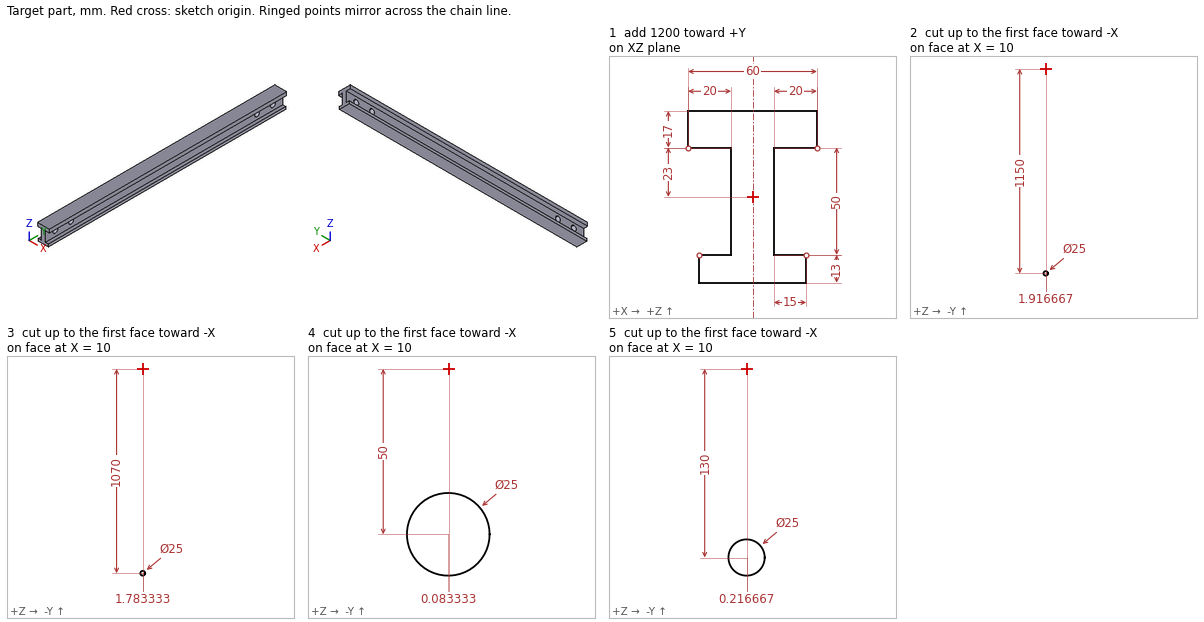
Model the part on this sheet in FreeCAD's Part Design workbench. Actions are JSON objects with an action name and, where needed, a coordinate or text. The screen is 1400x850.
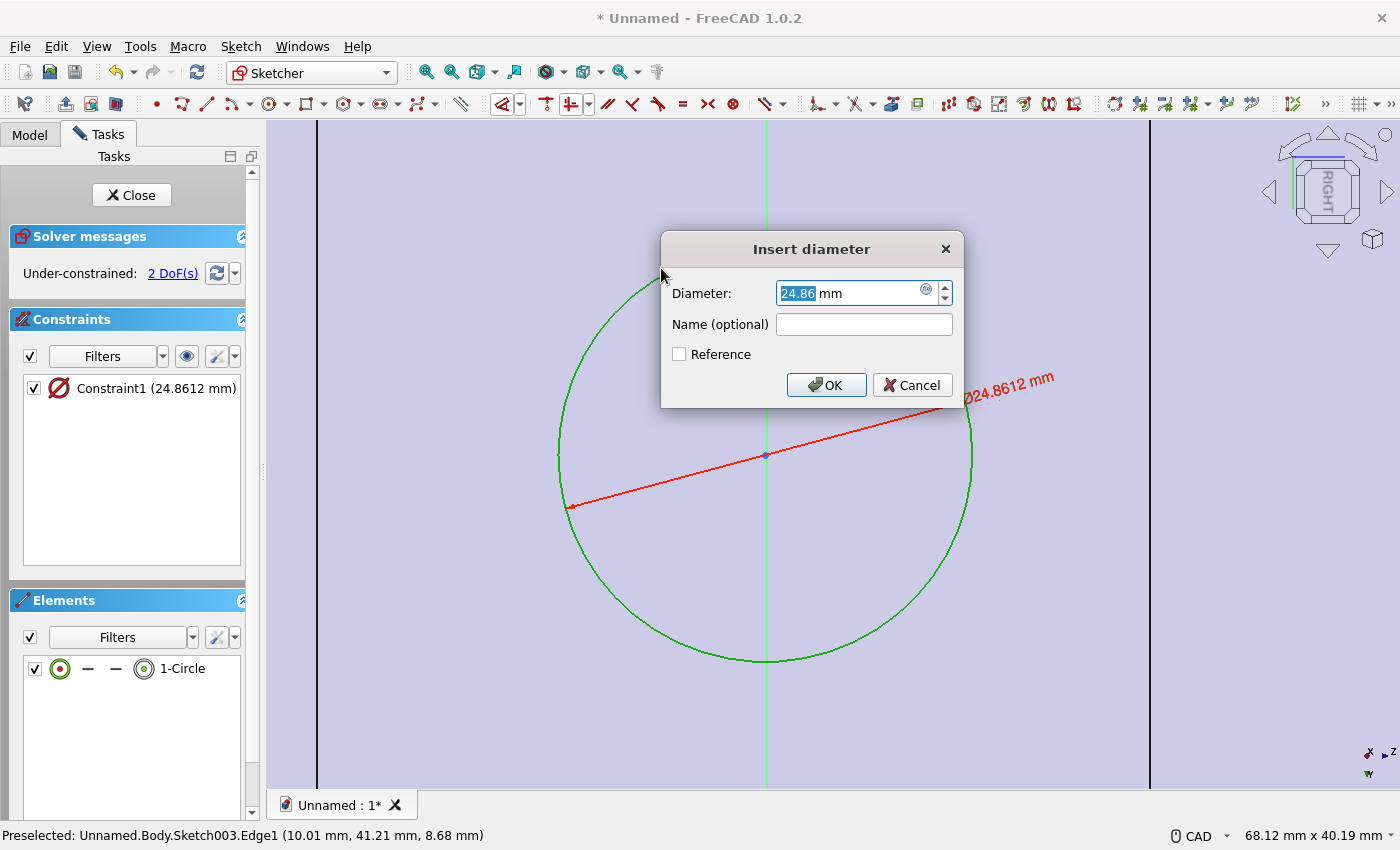
{"action": "type", "text": "25"}
{"action": "key", "text": "Return"}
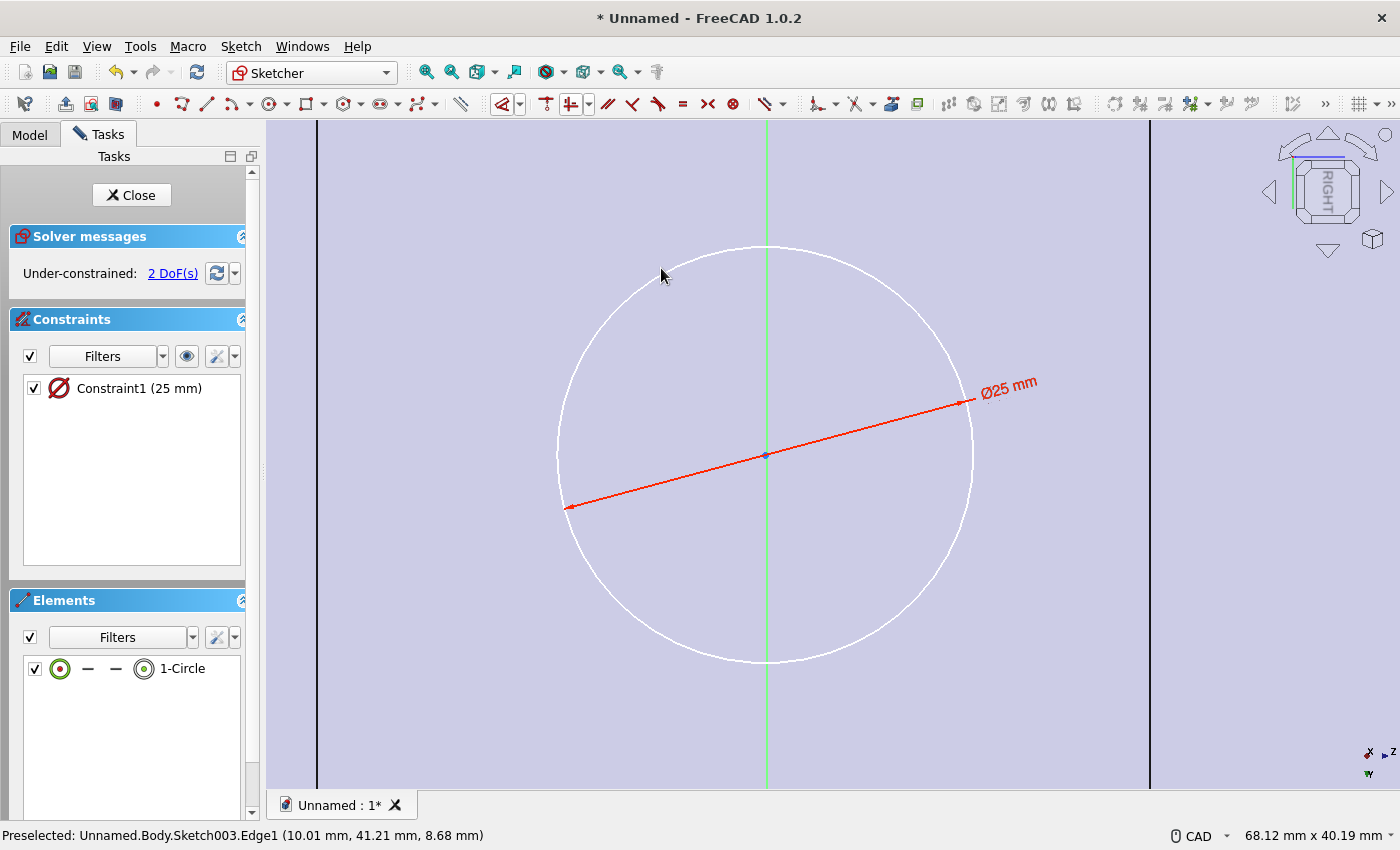
{"action": "left_click", "coordinate": [765, 455]}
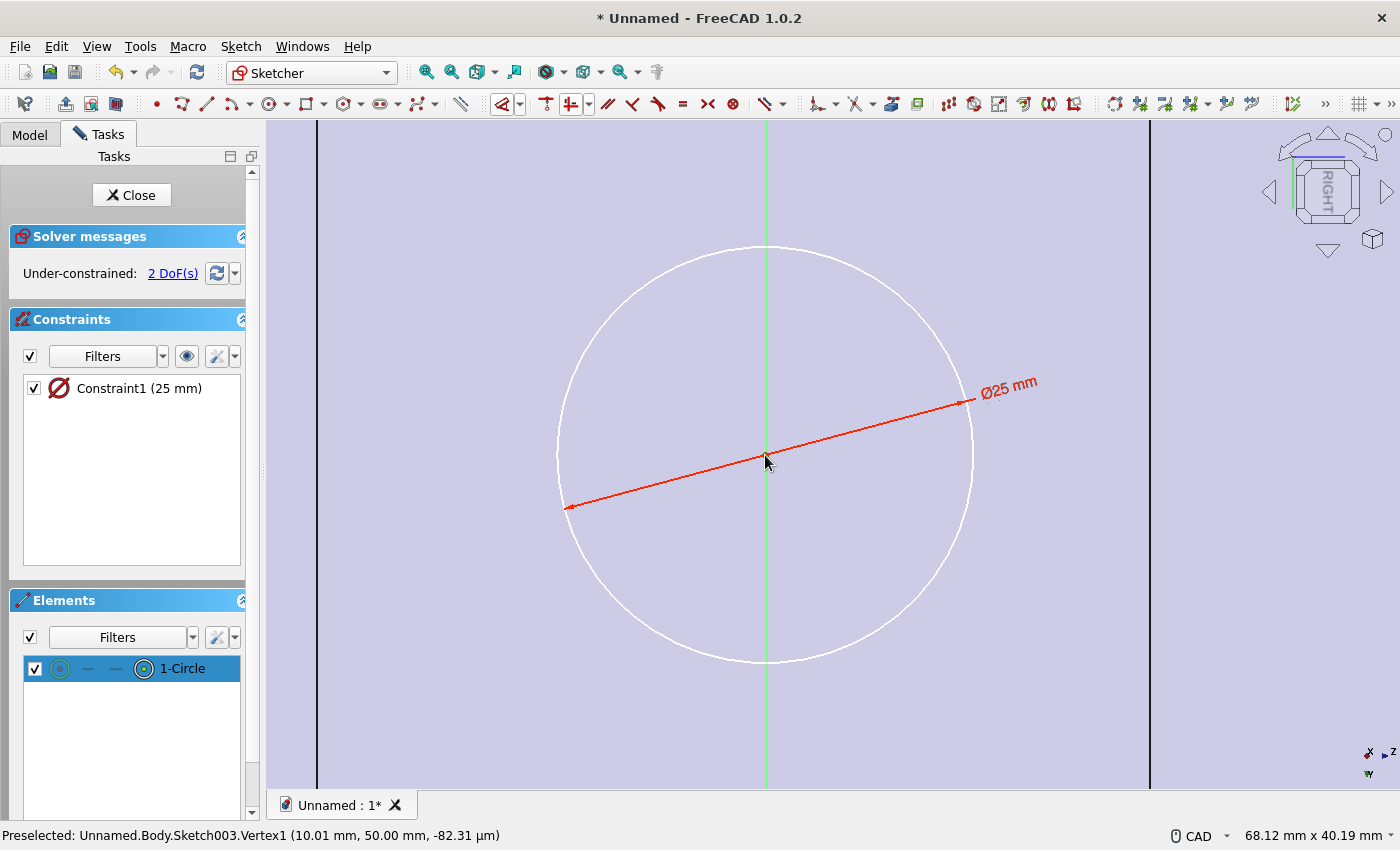
{"action": "left_click", "coordinate": [520, 104]}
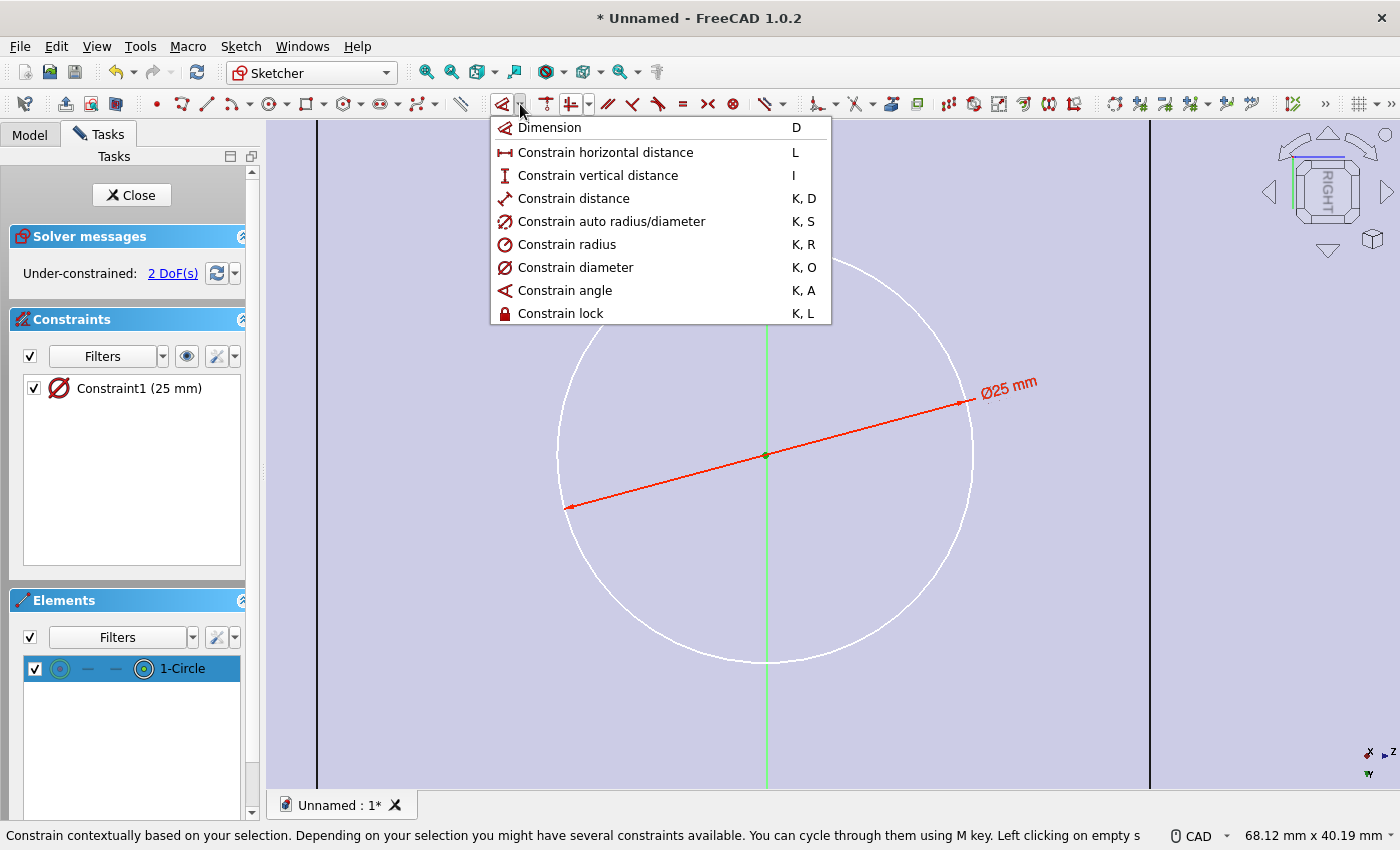
{"action": "left_click", "coordinate": [661, 176]}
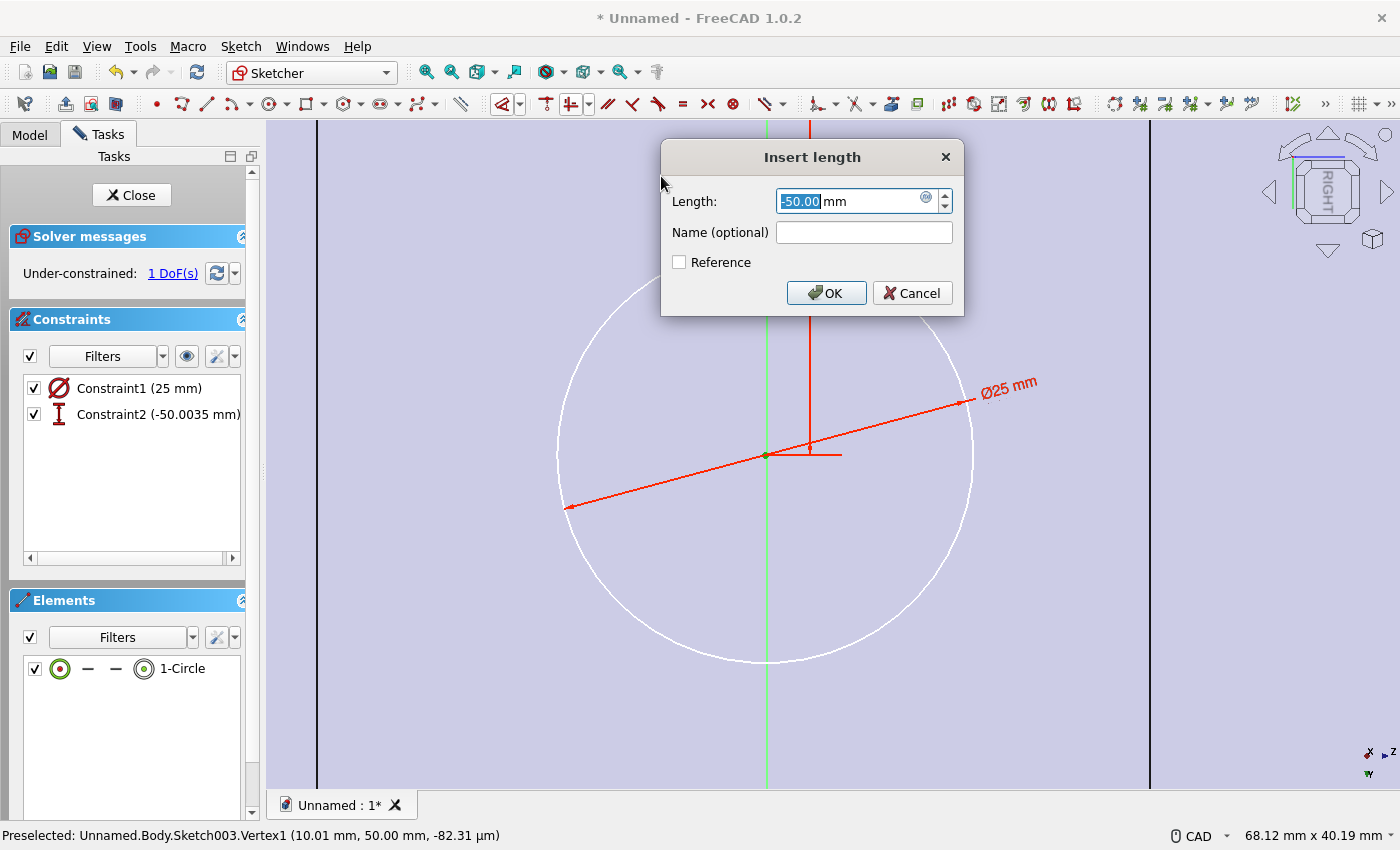
{"action": "type", "text": "-50"}
{"action": "key", "text": "Return"}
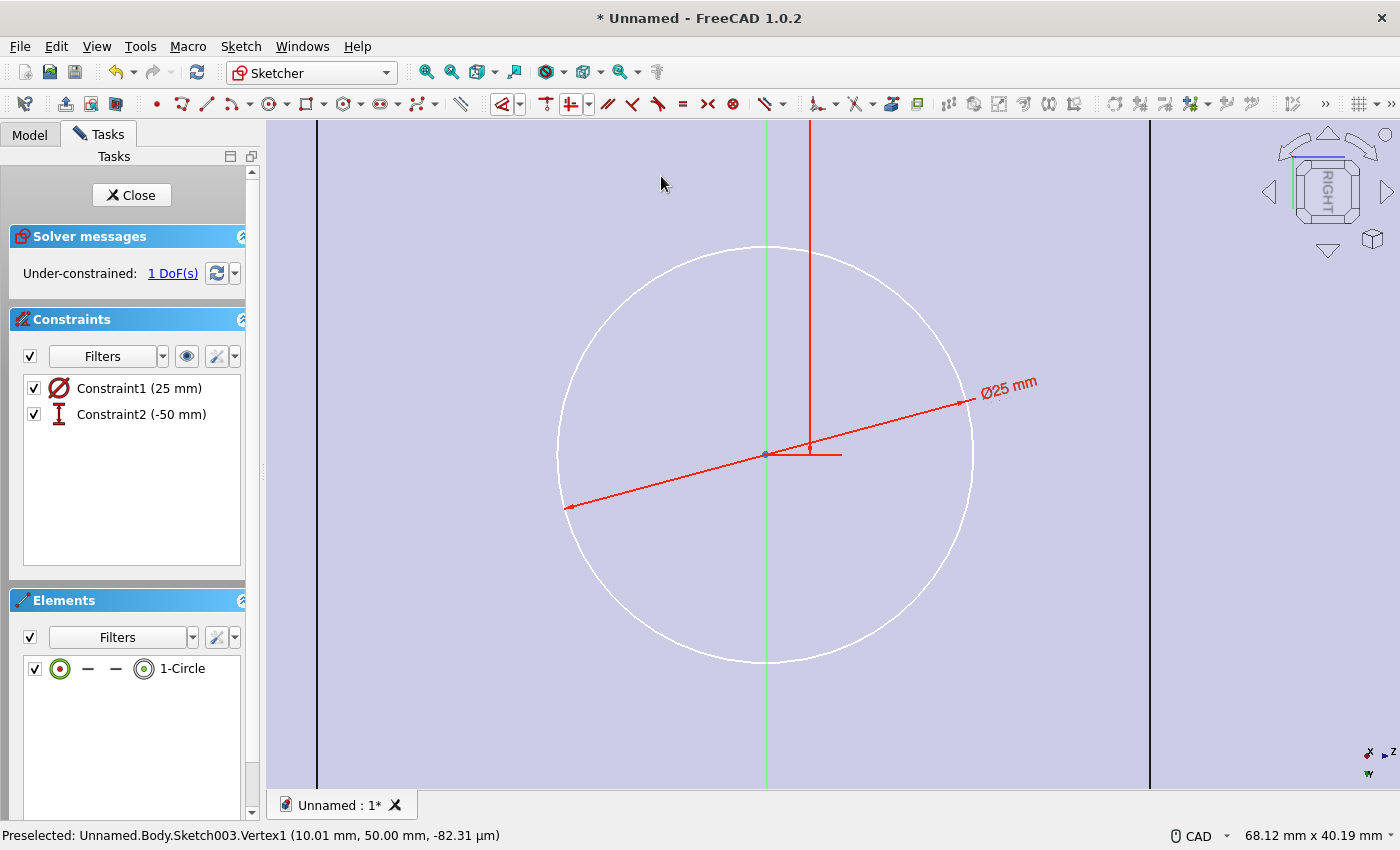
{"action": "scroll", "coordinate": [765, 455], "scroll_direction": "up", "scroll_amount": 17}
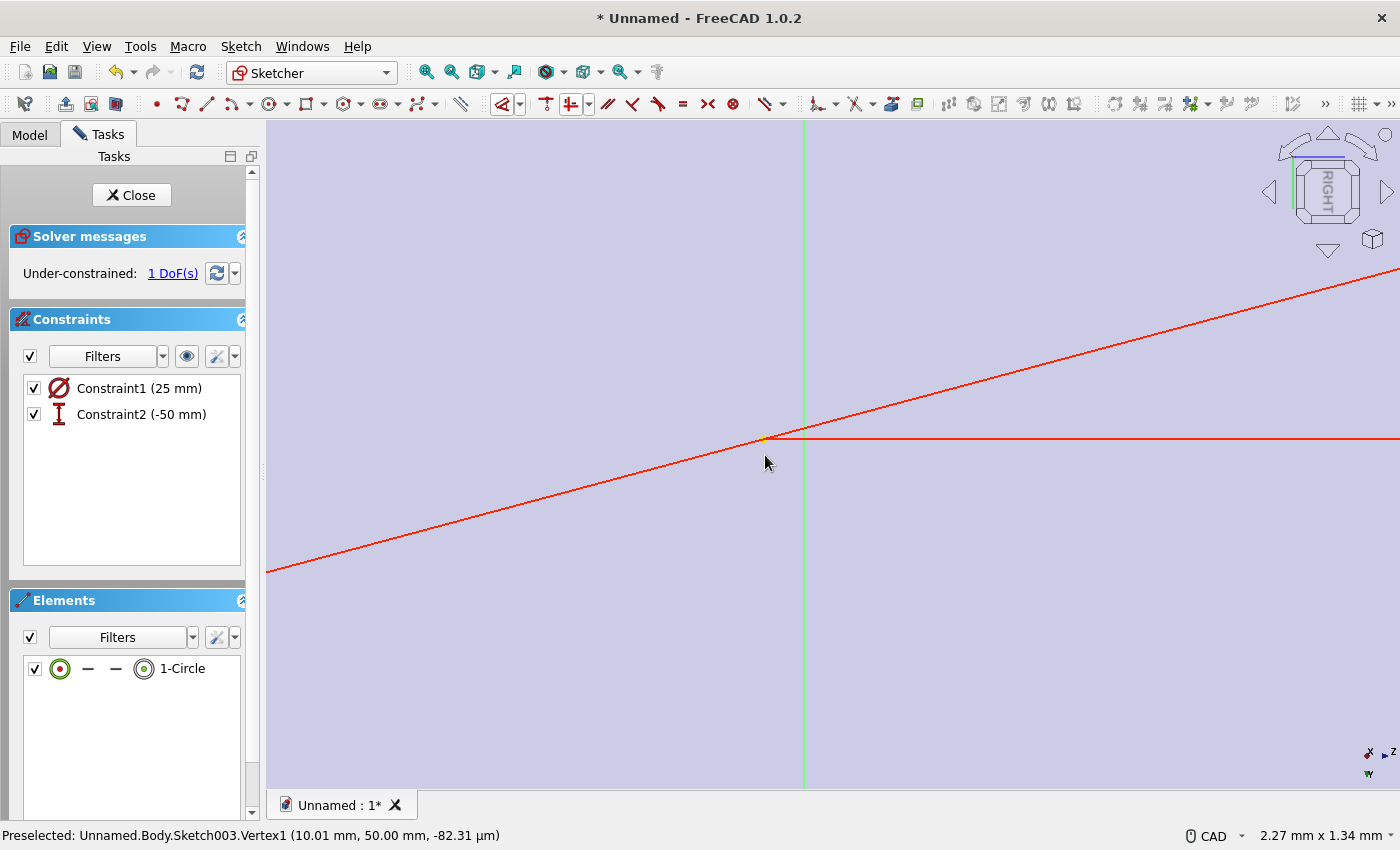
{"action": "left_click", "coordinate": [763, 439]}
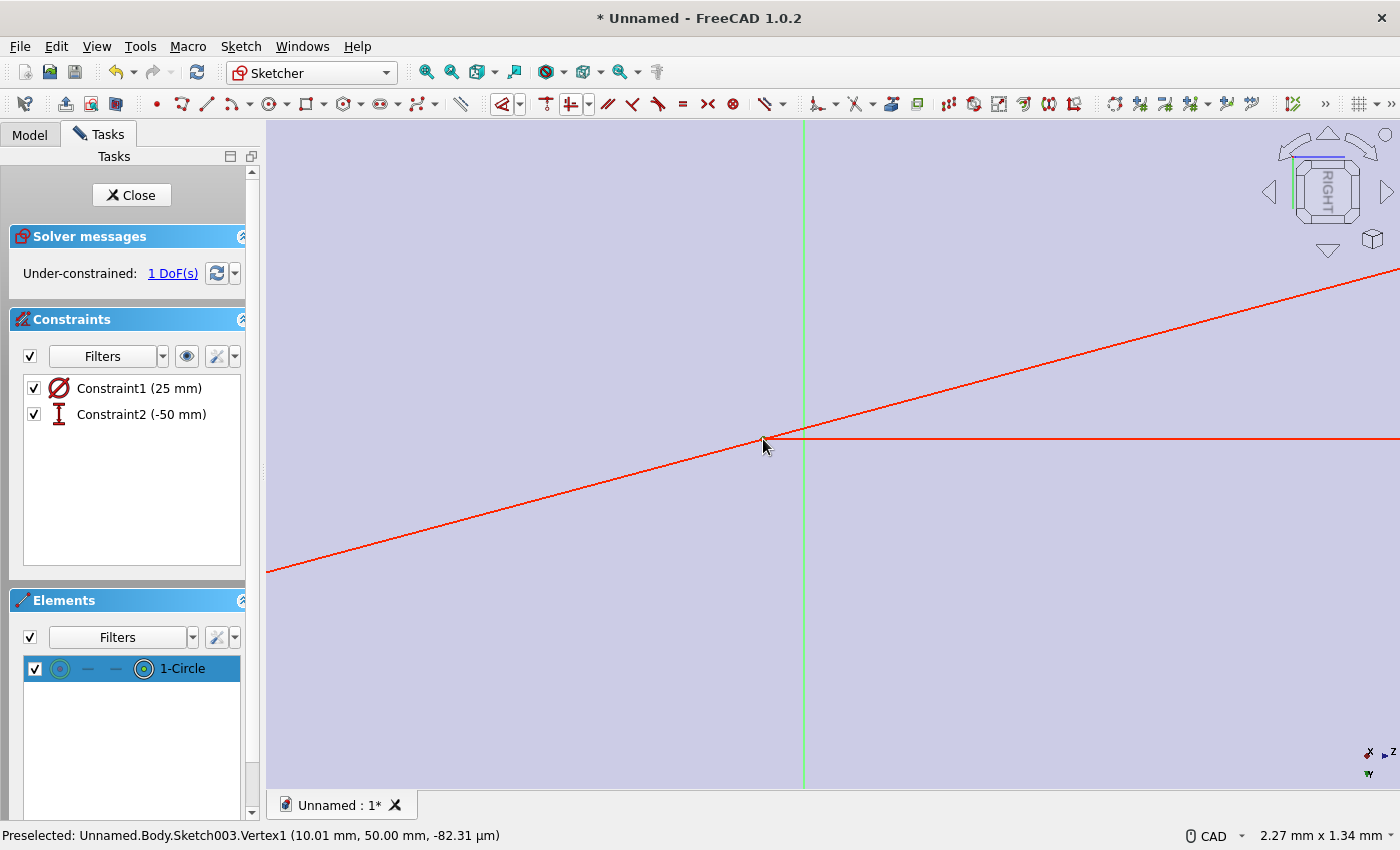
{"action": "key", "text": "l"}